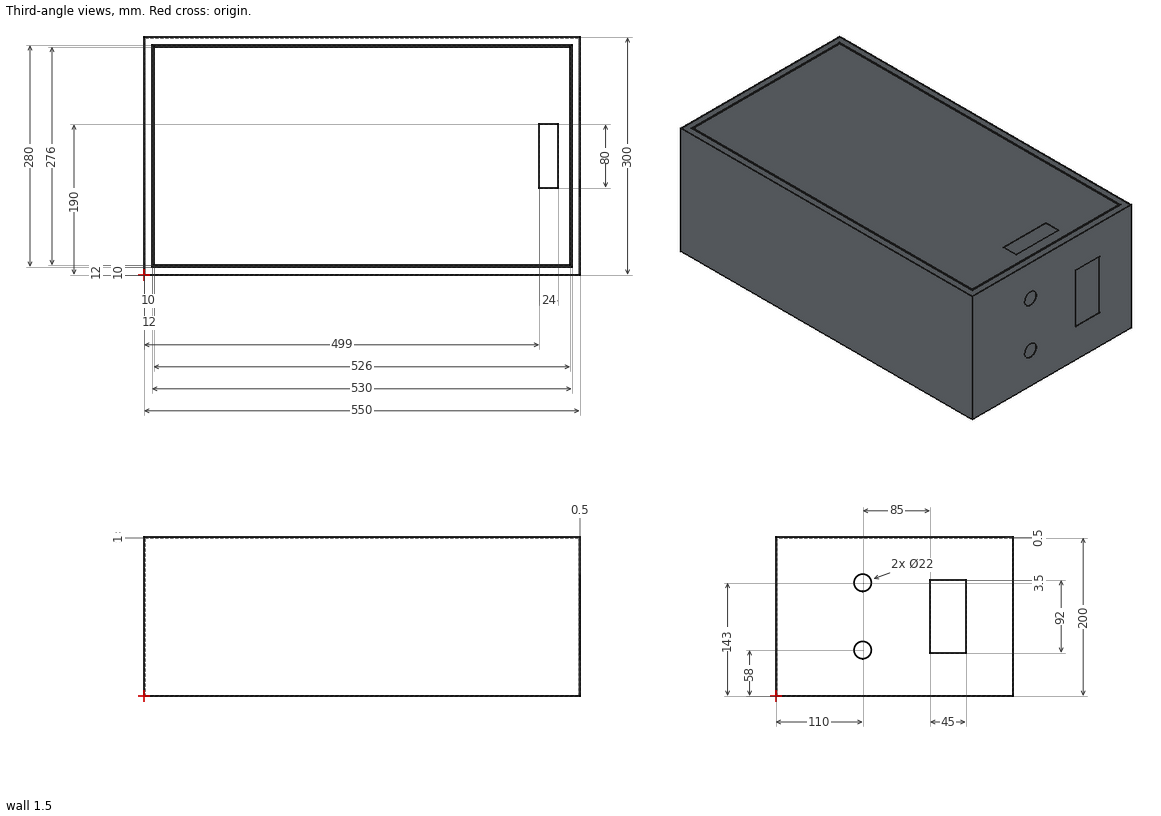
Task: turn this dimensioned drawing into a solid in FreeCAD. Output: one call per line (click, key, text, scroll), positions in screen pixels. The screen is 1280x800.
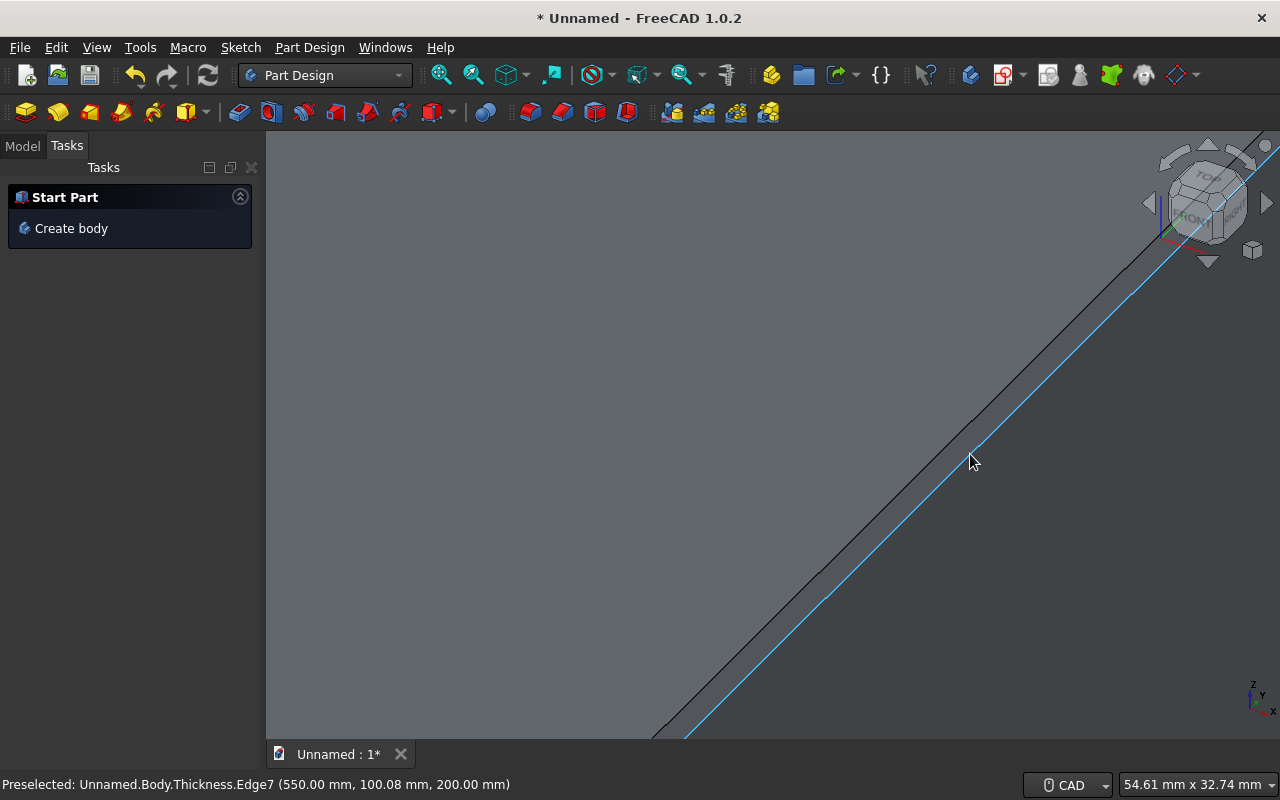
click(442, 76)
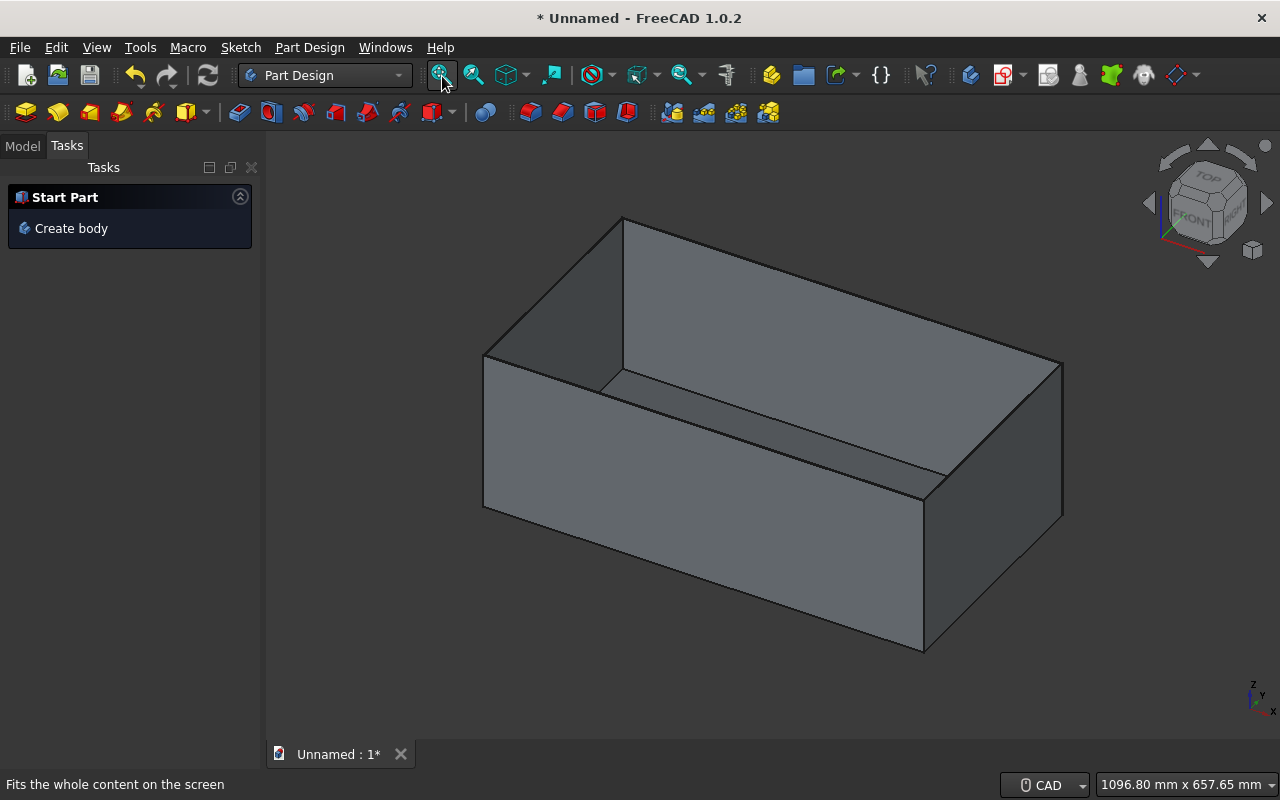
key(0)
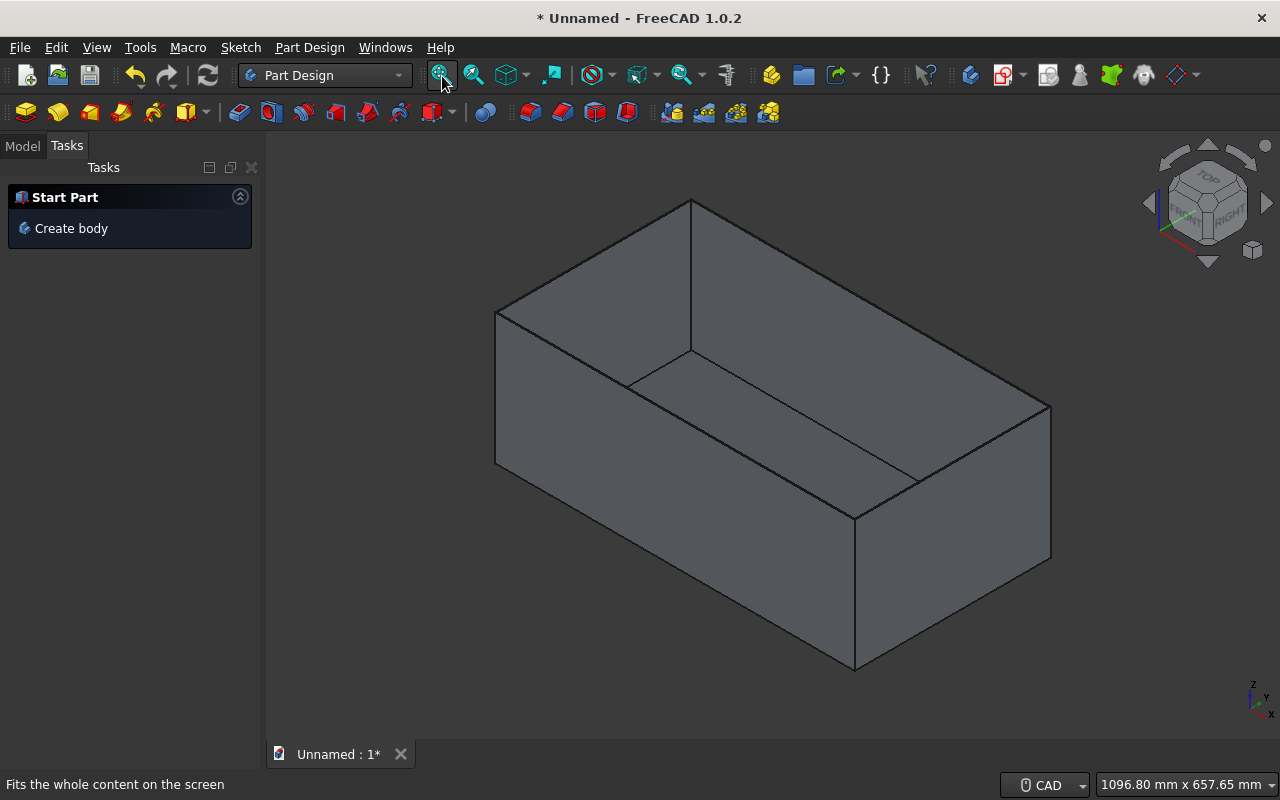
scroll(920, 481, up, 15)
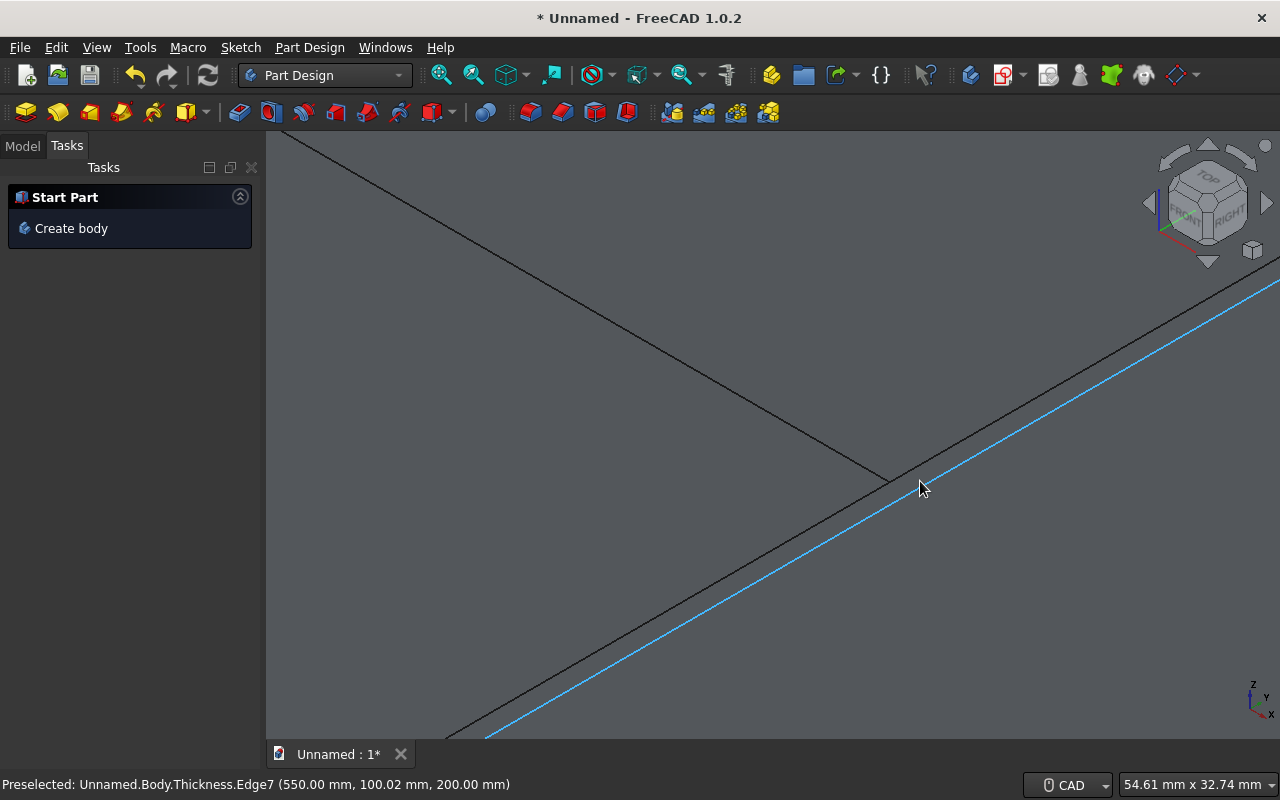
click(442, 76)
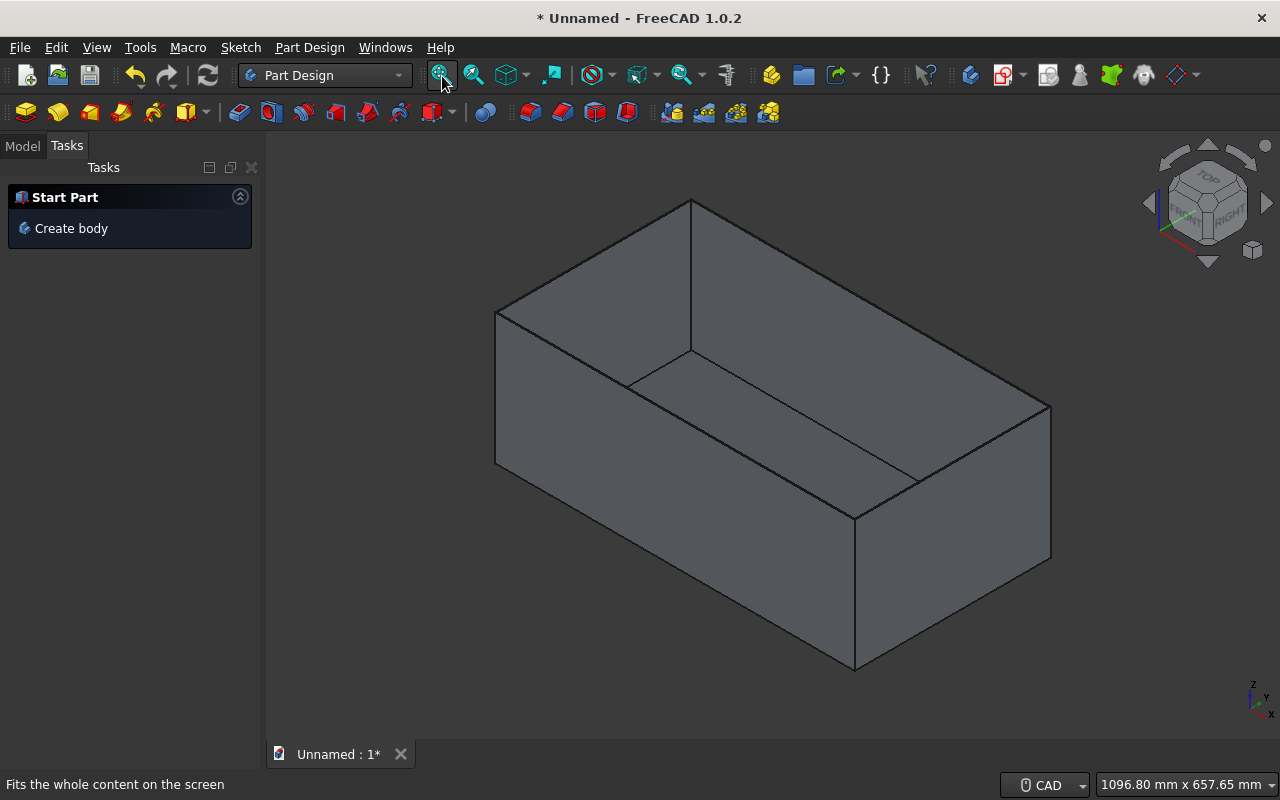
key(2)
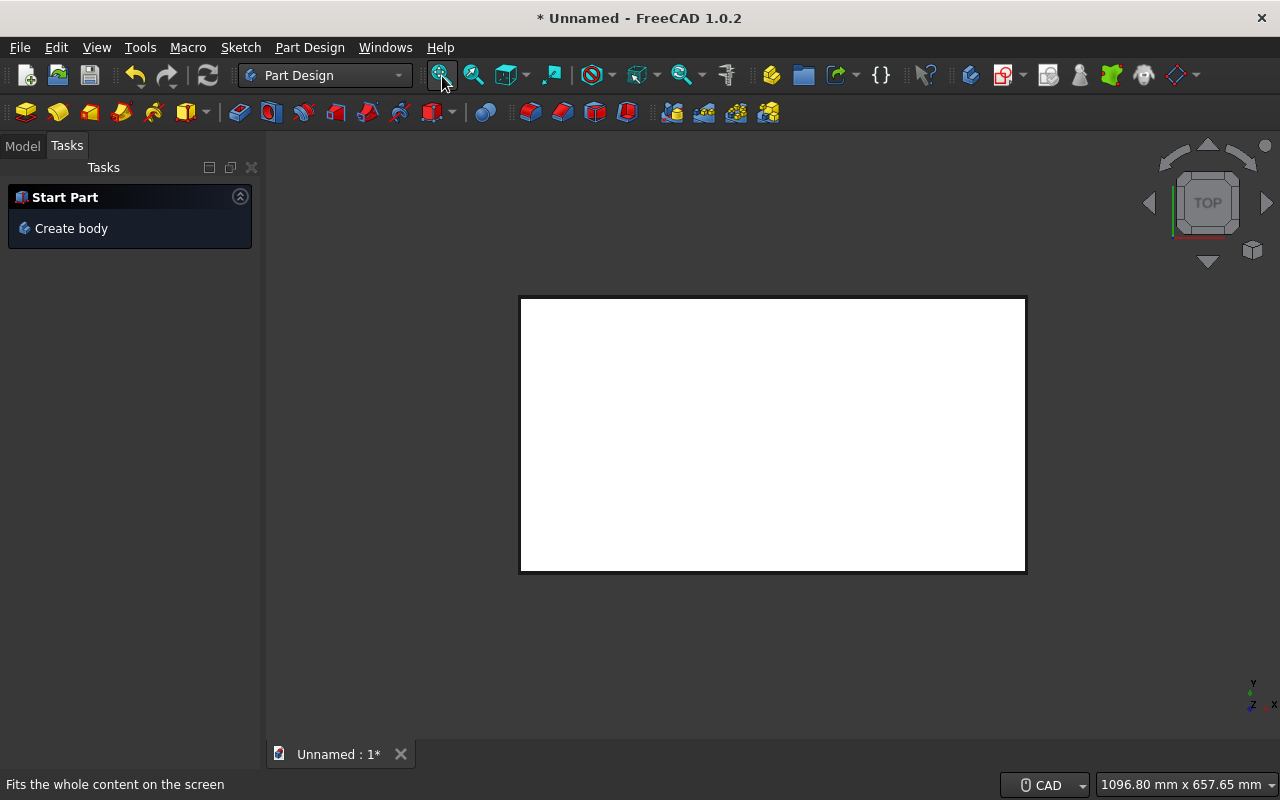
scroll(1027, 480, up, 15)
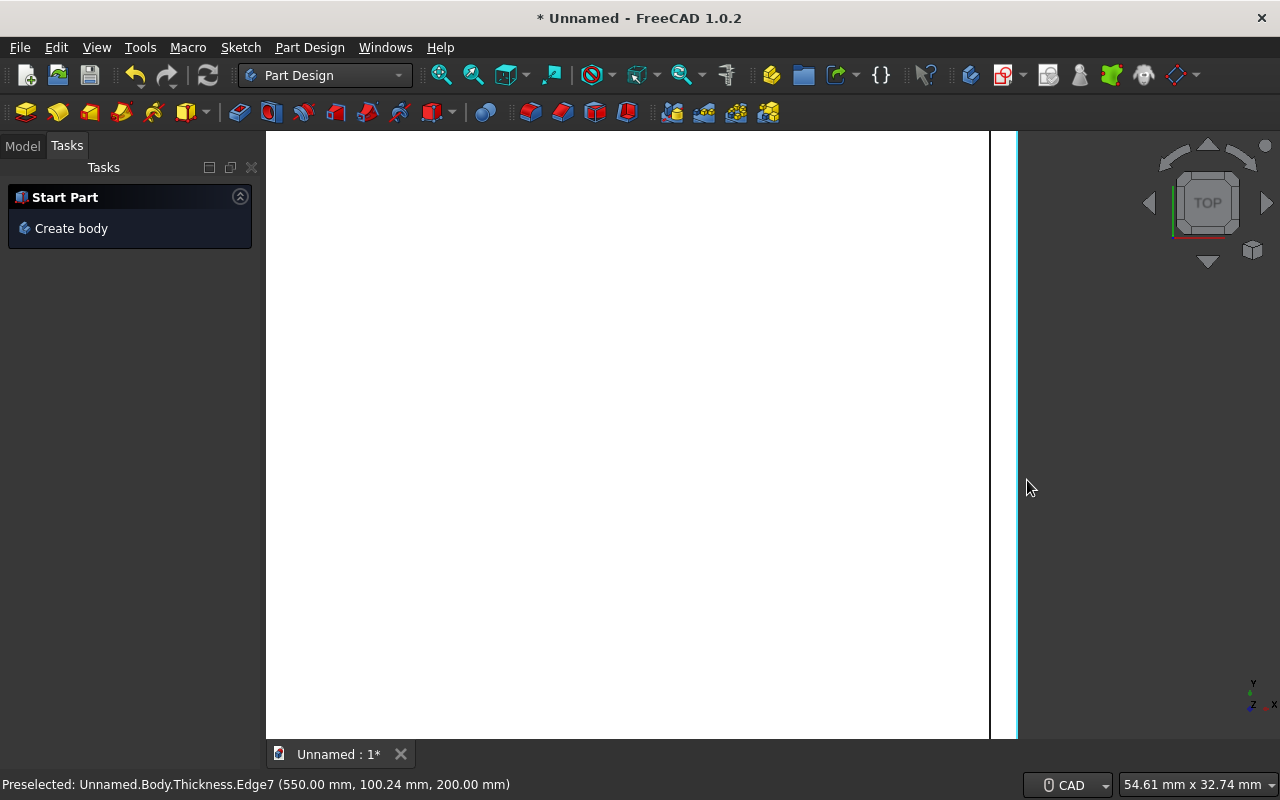
click(1008, 483)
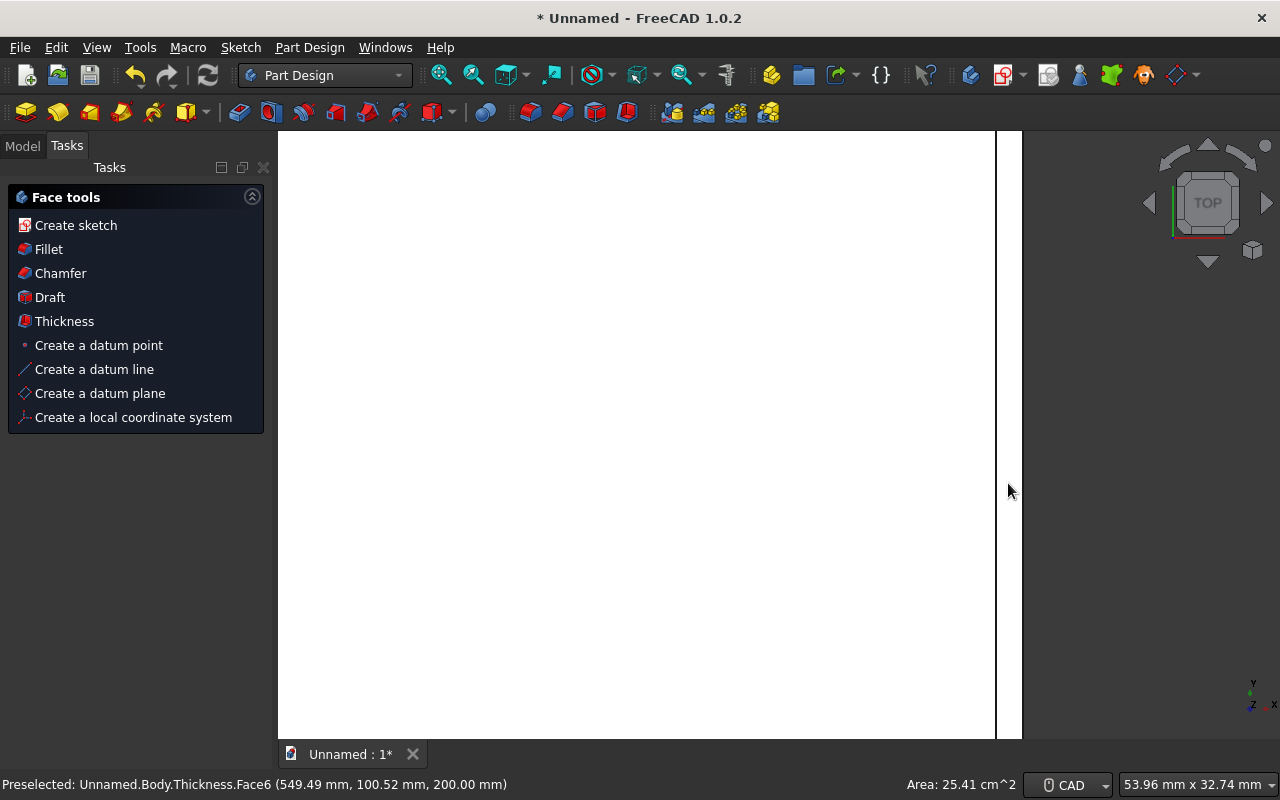
click(1004, 76)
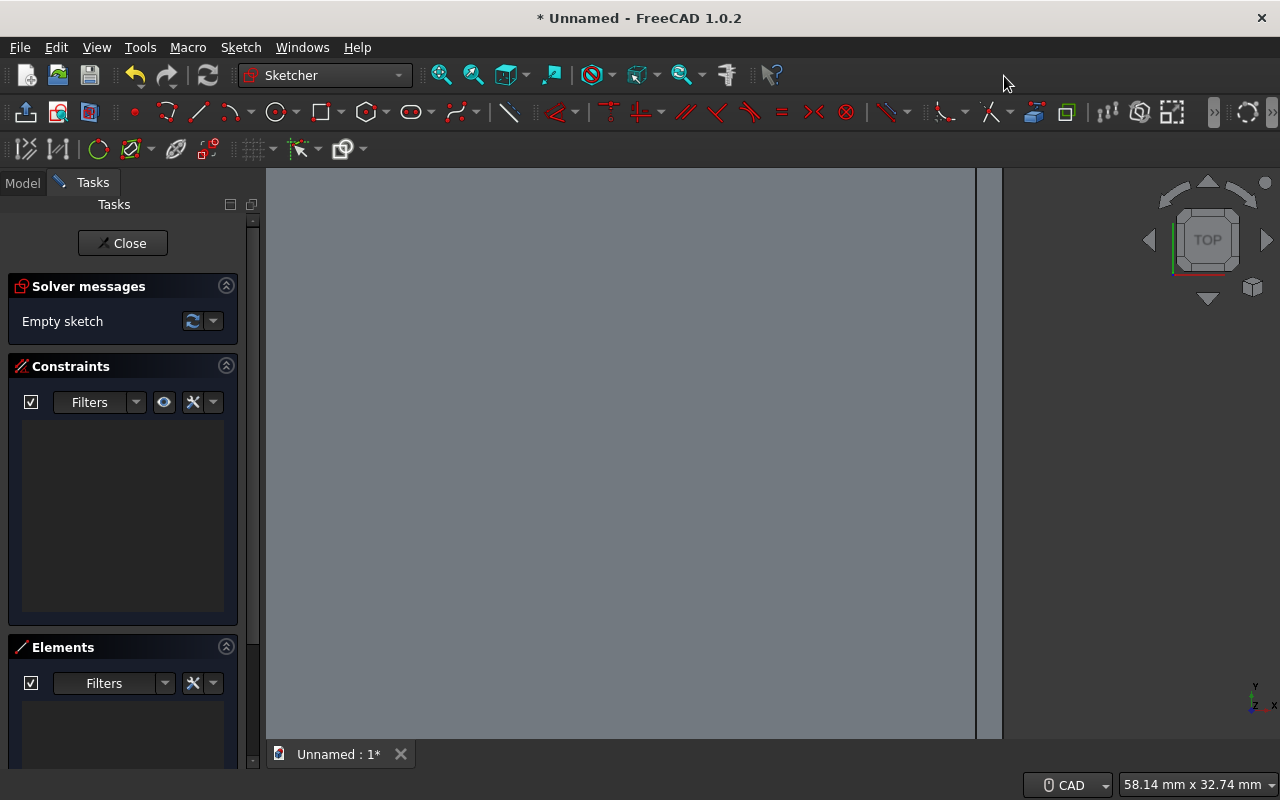
scroll(996, 506, down, 14)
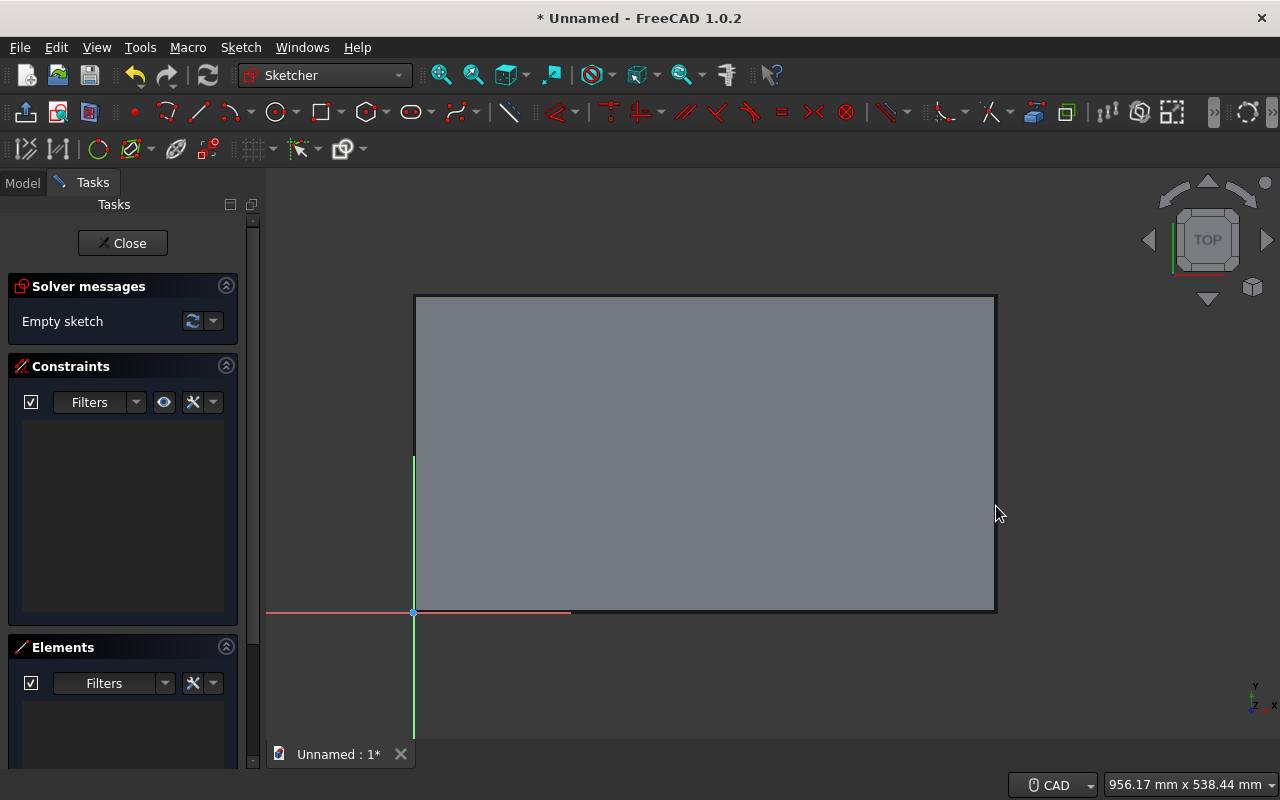
click(322, 112)